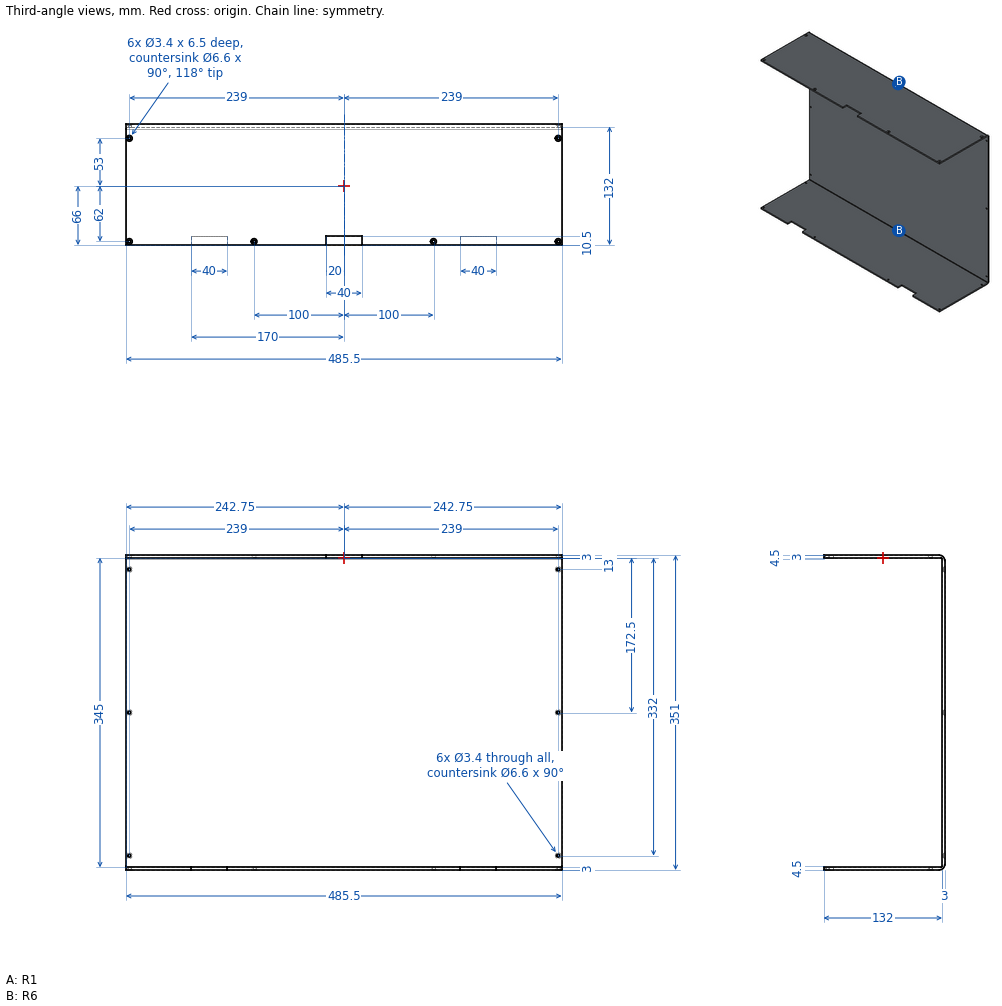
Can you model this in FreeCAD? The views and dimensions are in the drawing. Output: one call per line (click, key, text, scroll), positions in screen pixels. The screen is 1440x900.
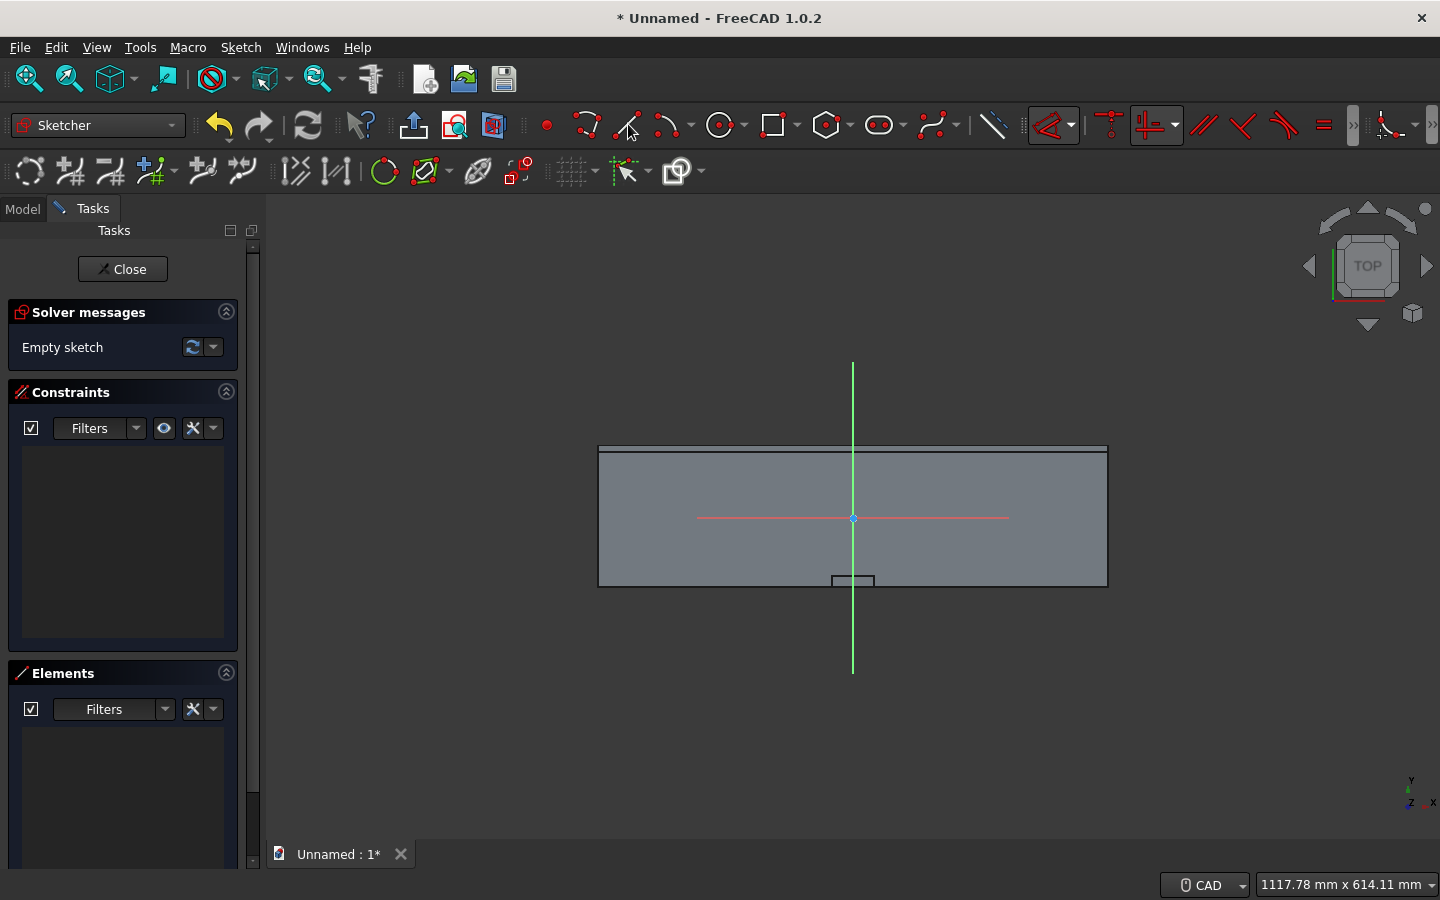
scroll(992, 536, up, 2)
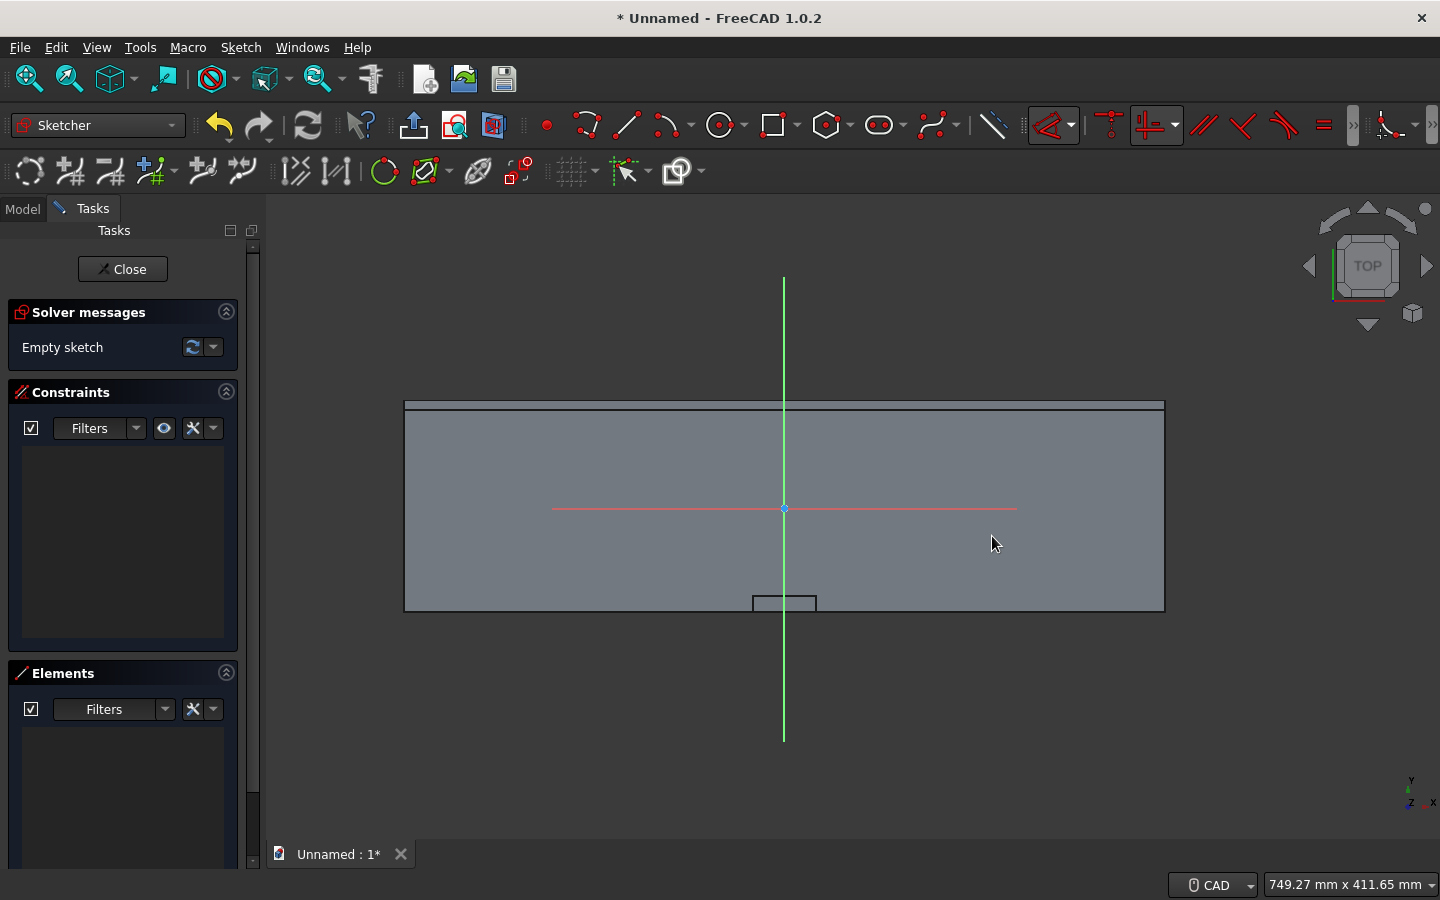
click(720, 126)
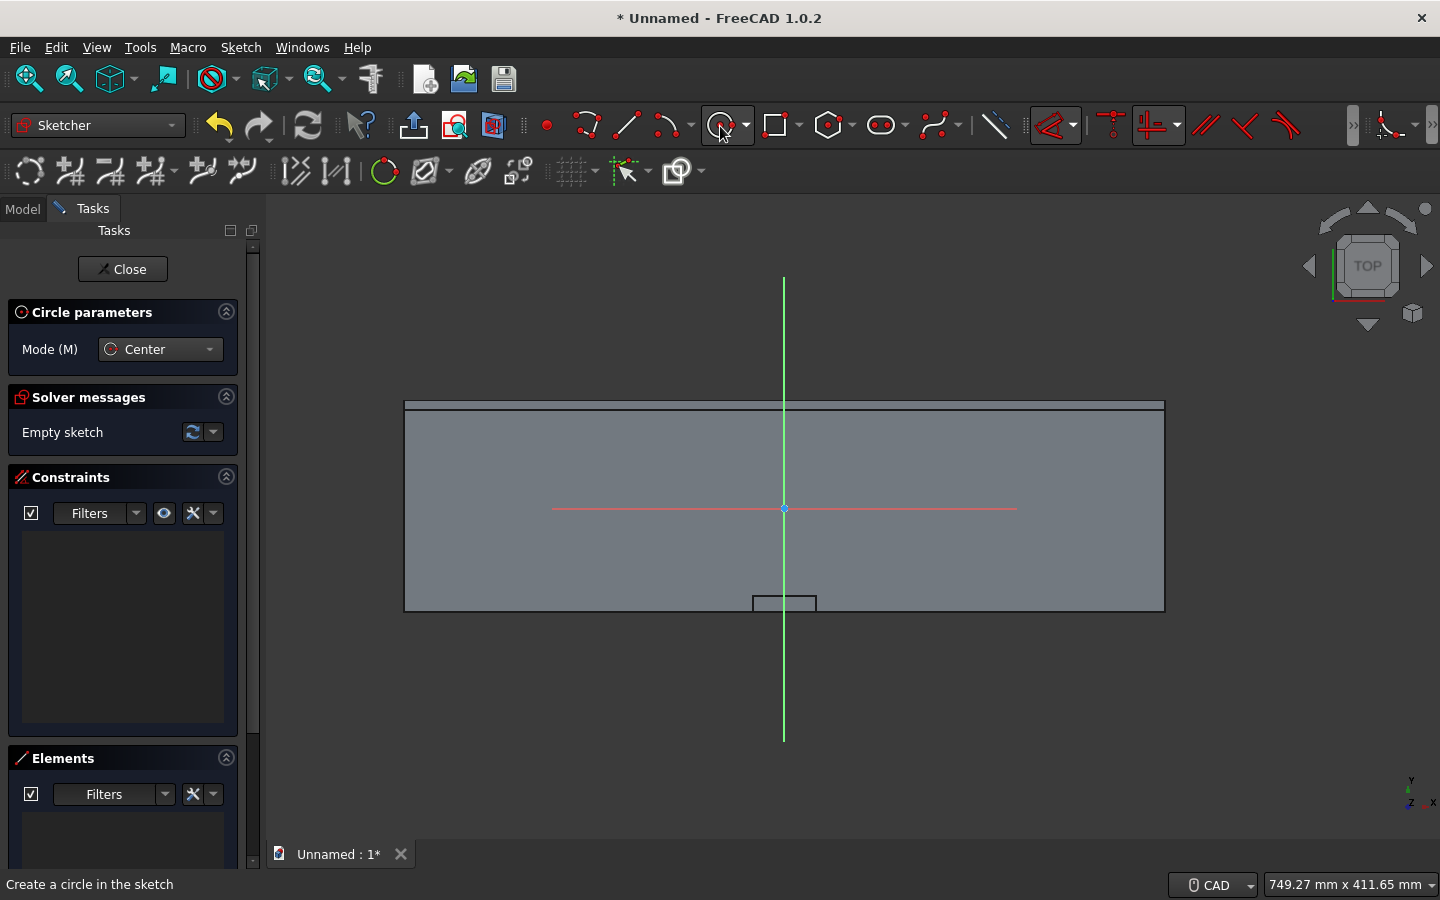
scroll(410, 426, up, 11)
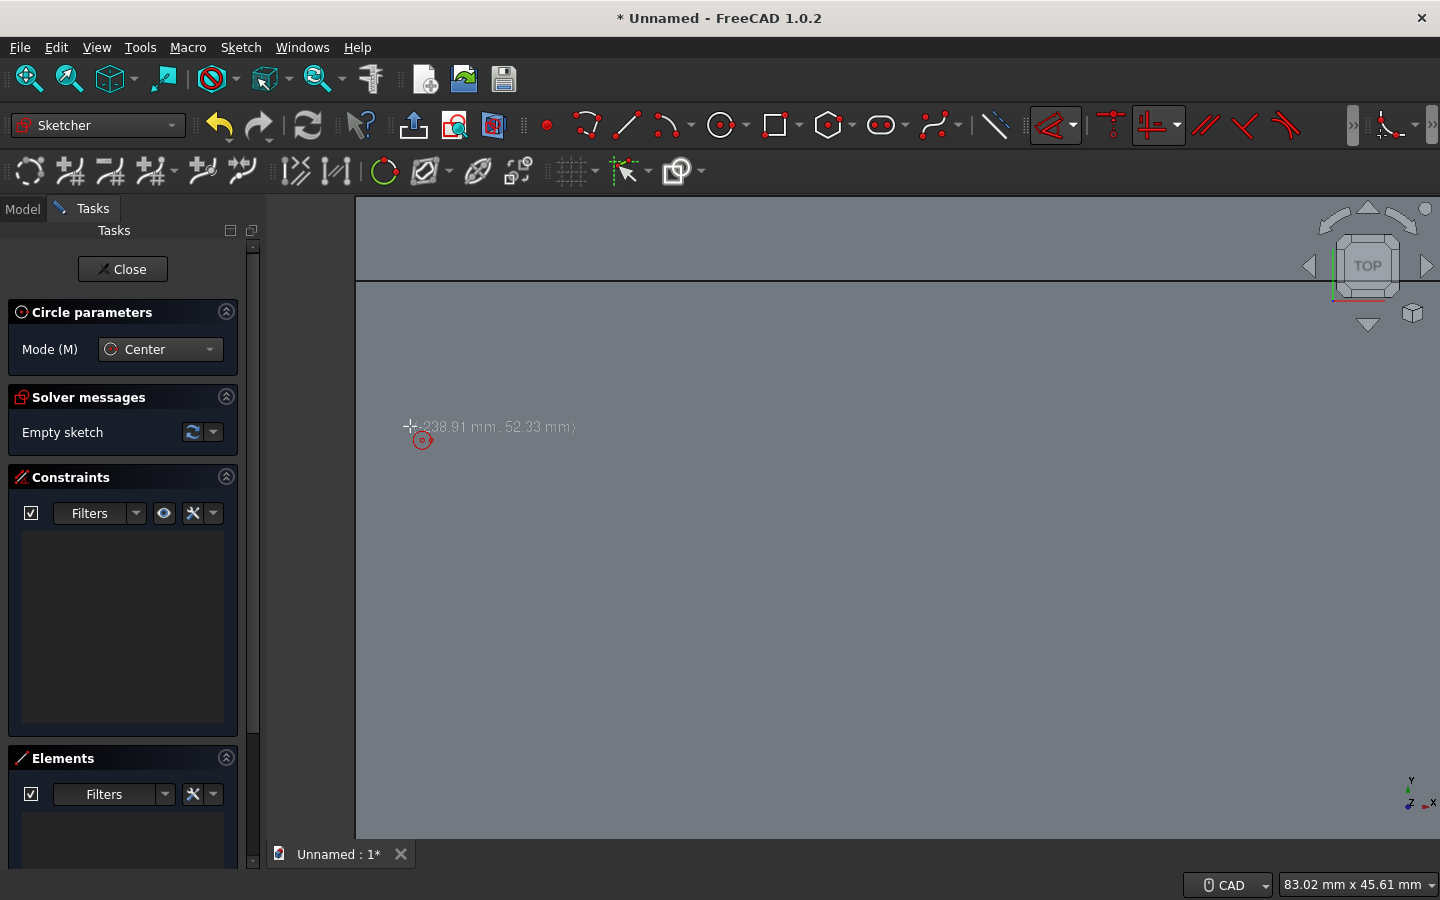
scroll(410, 427, down, 11)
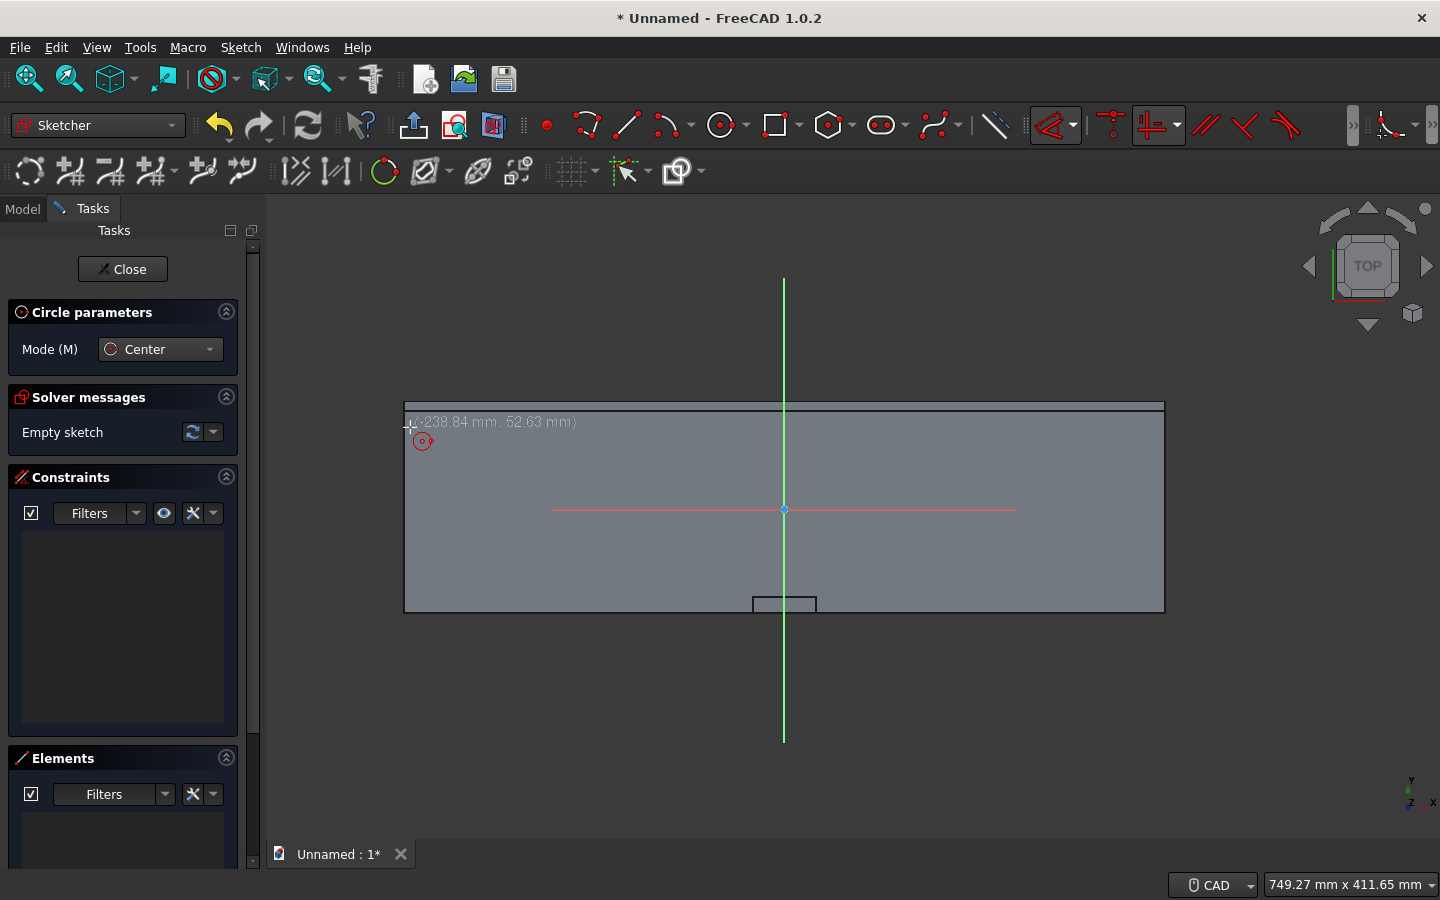
click(410, 427)
move(412, 425)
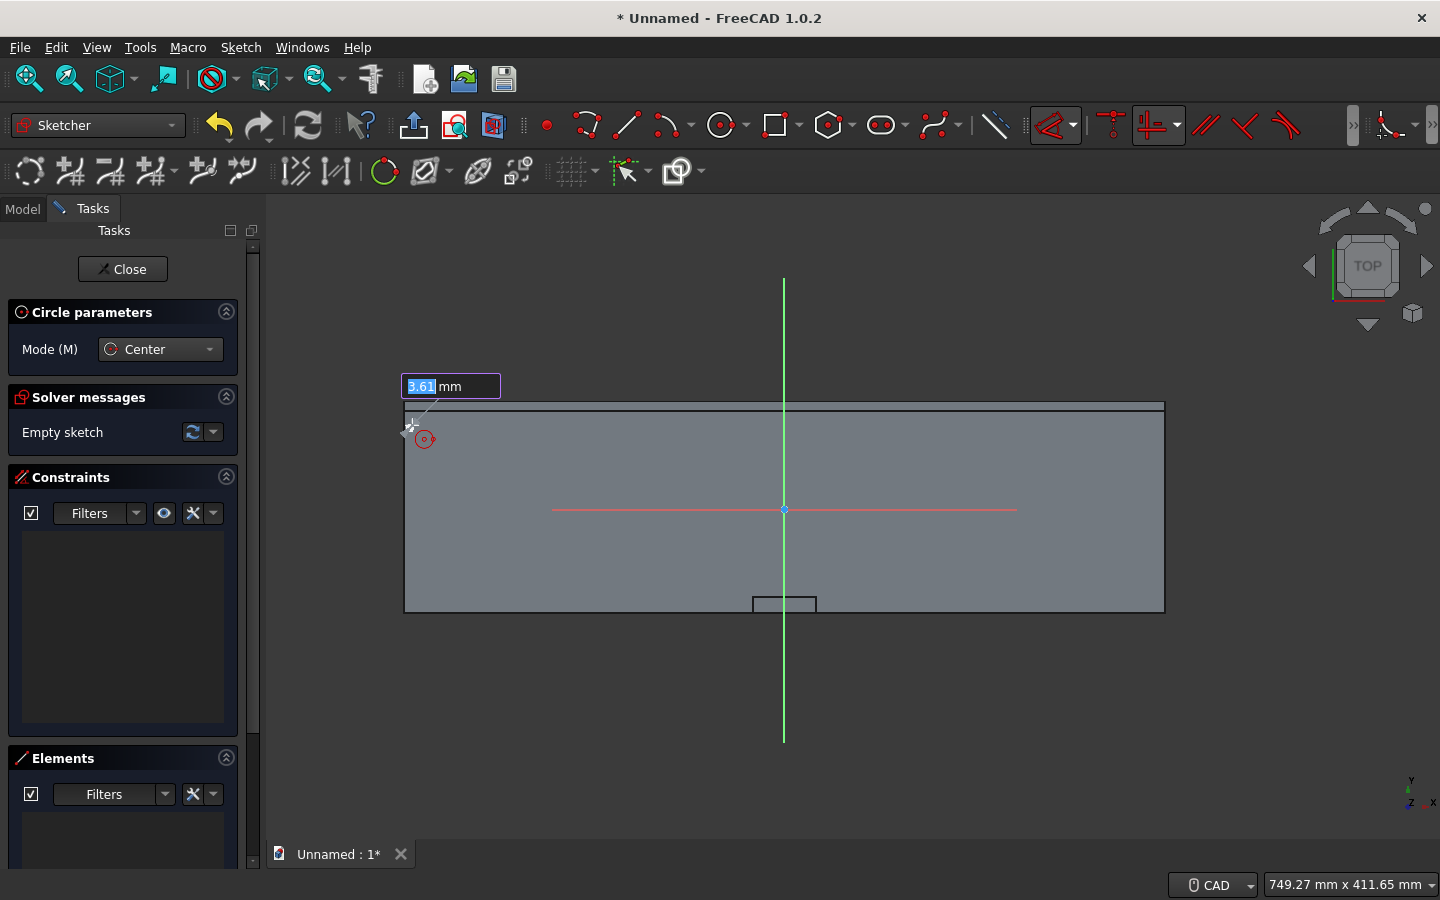
text(3.4)
key(Return)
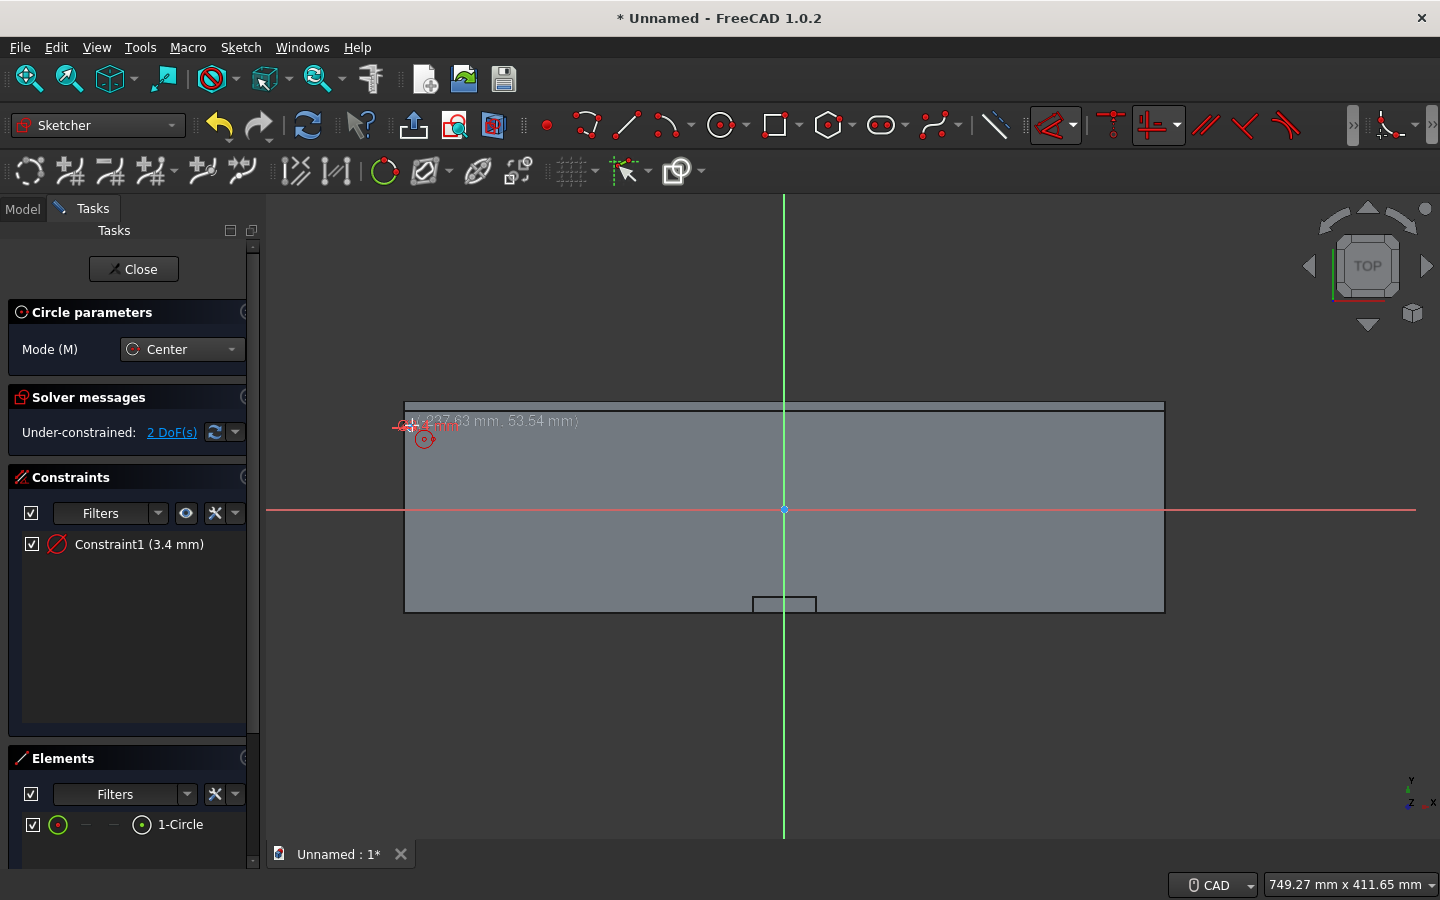
scroll(410, 607, up, 11)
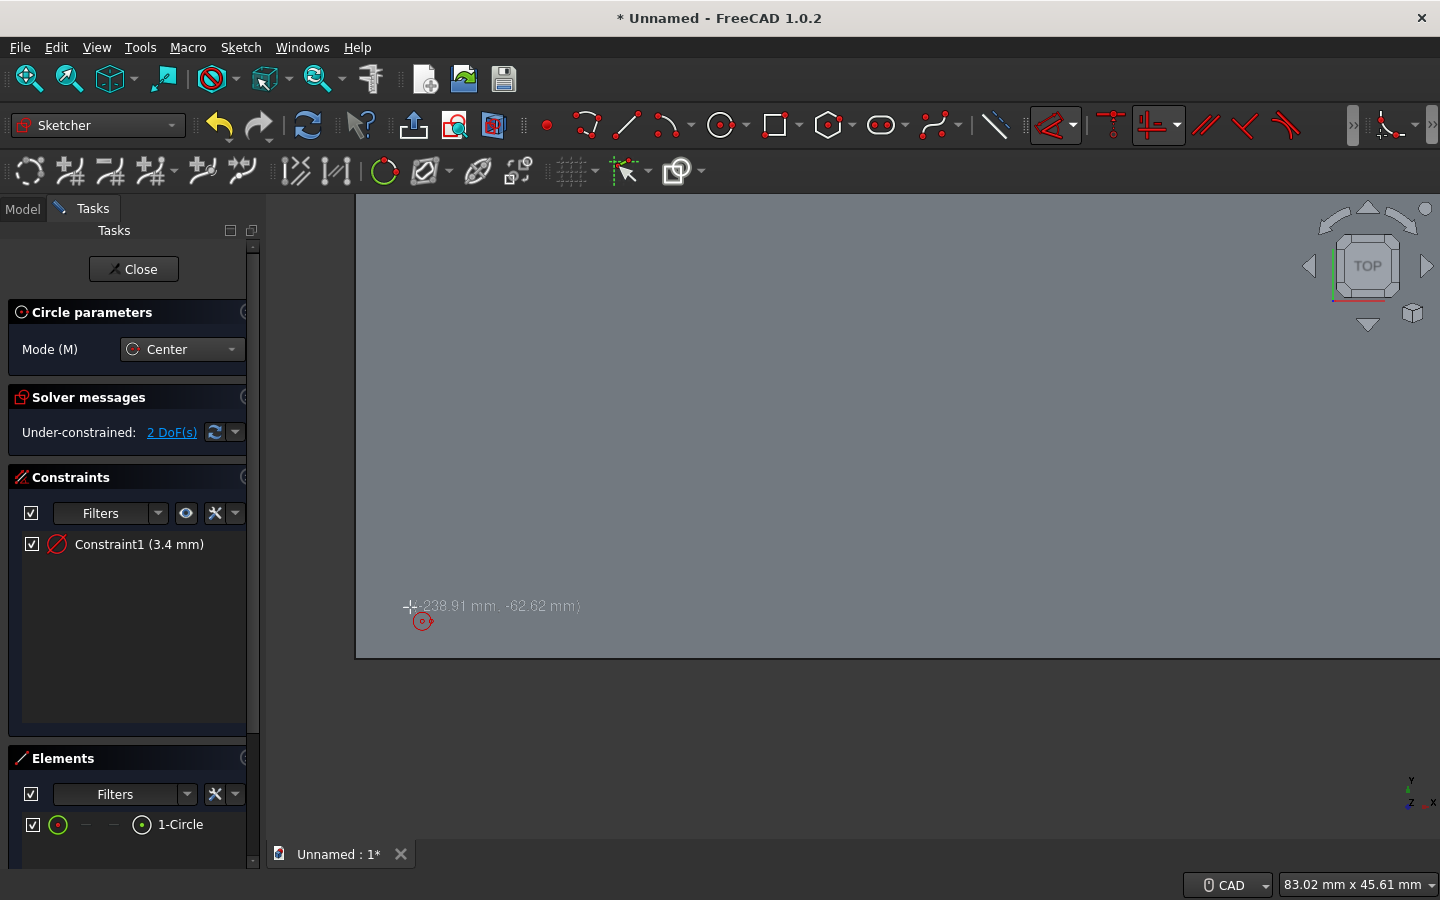
scroll(410, 607, down, 11)